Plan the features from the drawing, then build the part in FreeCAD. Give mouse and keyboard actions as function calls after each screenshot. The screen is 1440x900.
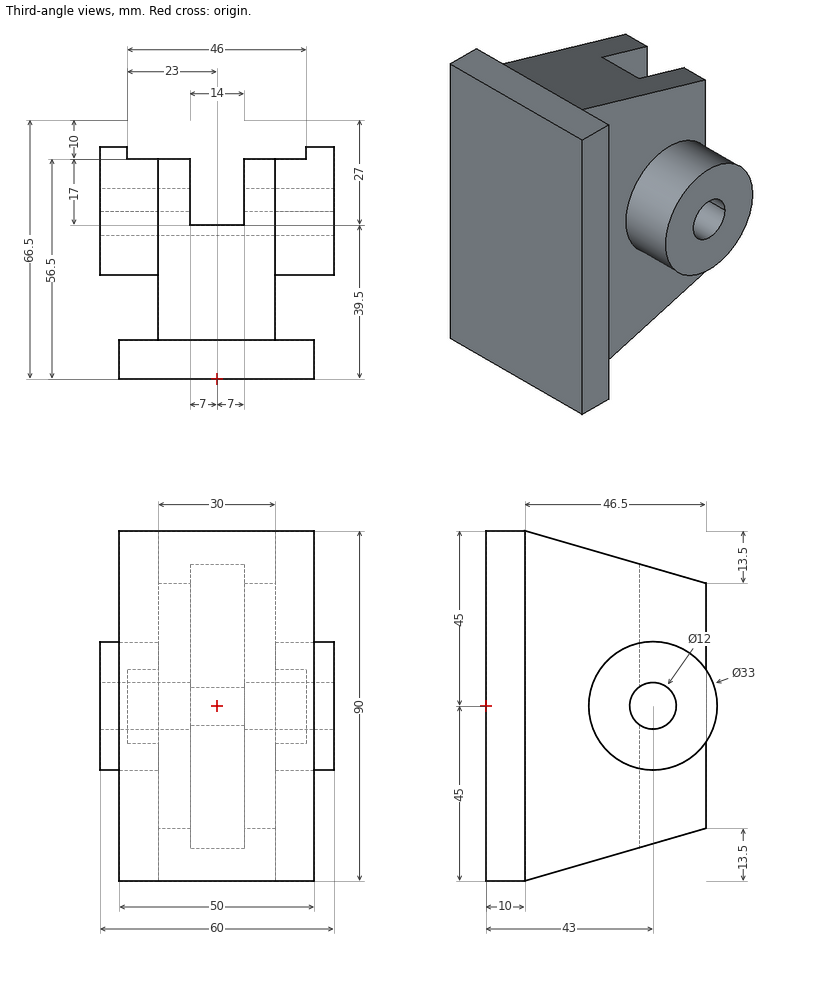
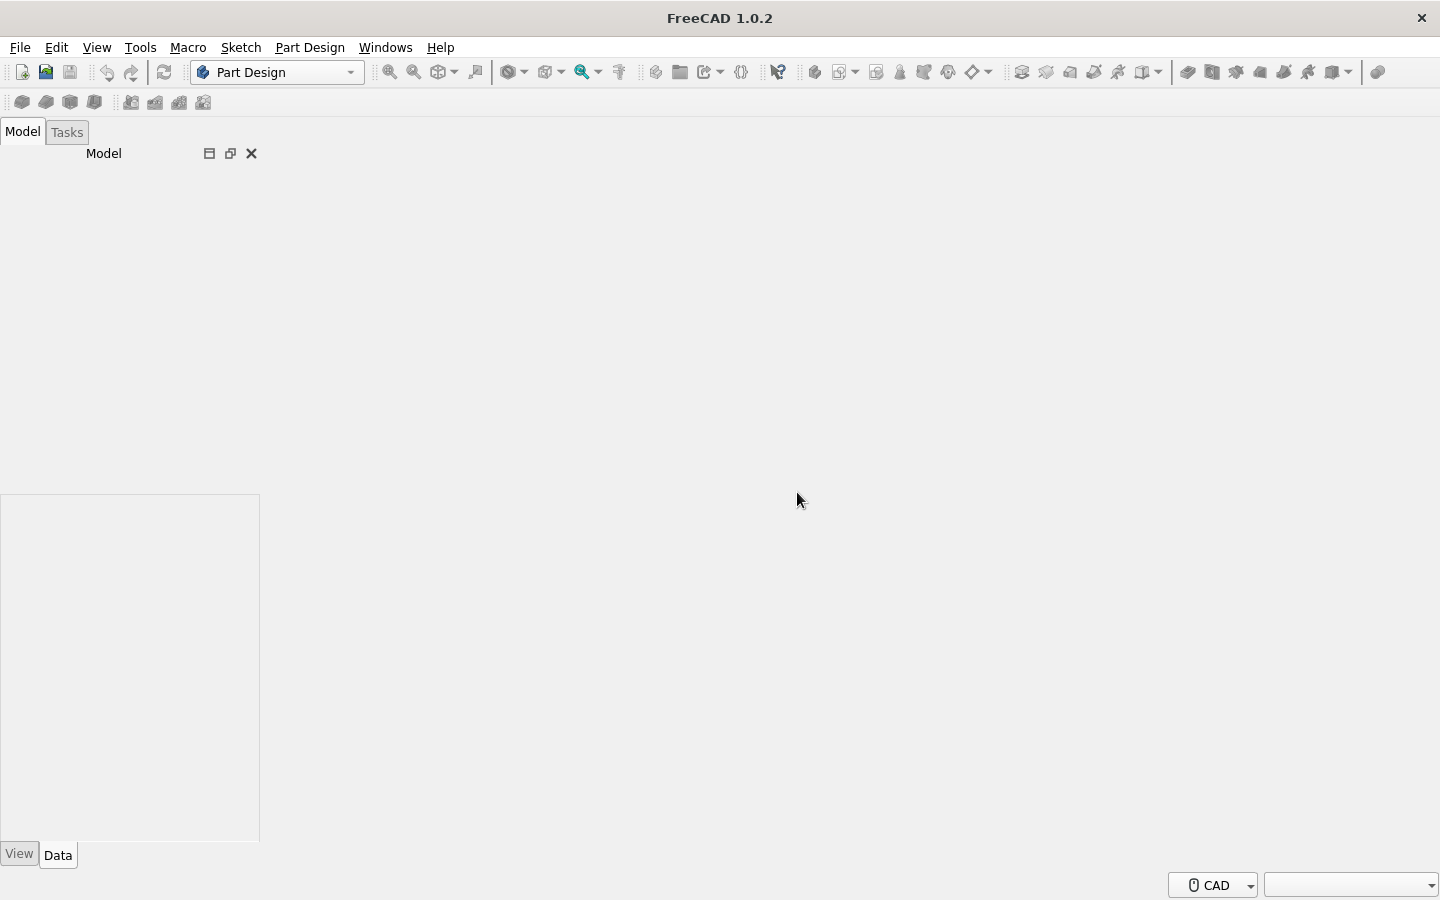
click(22, 72)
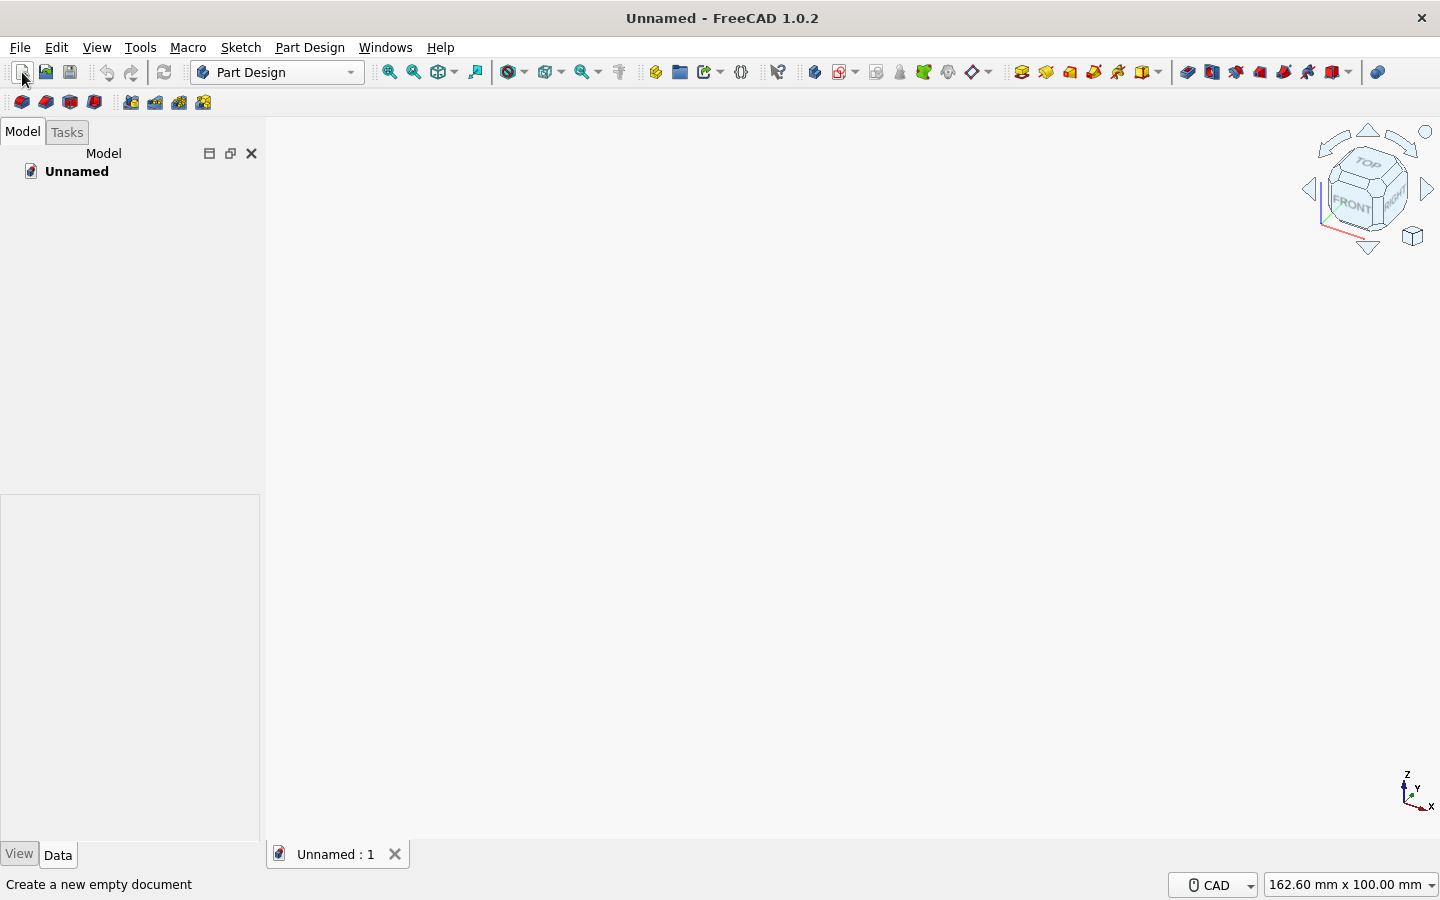
click(840, 72)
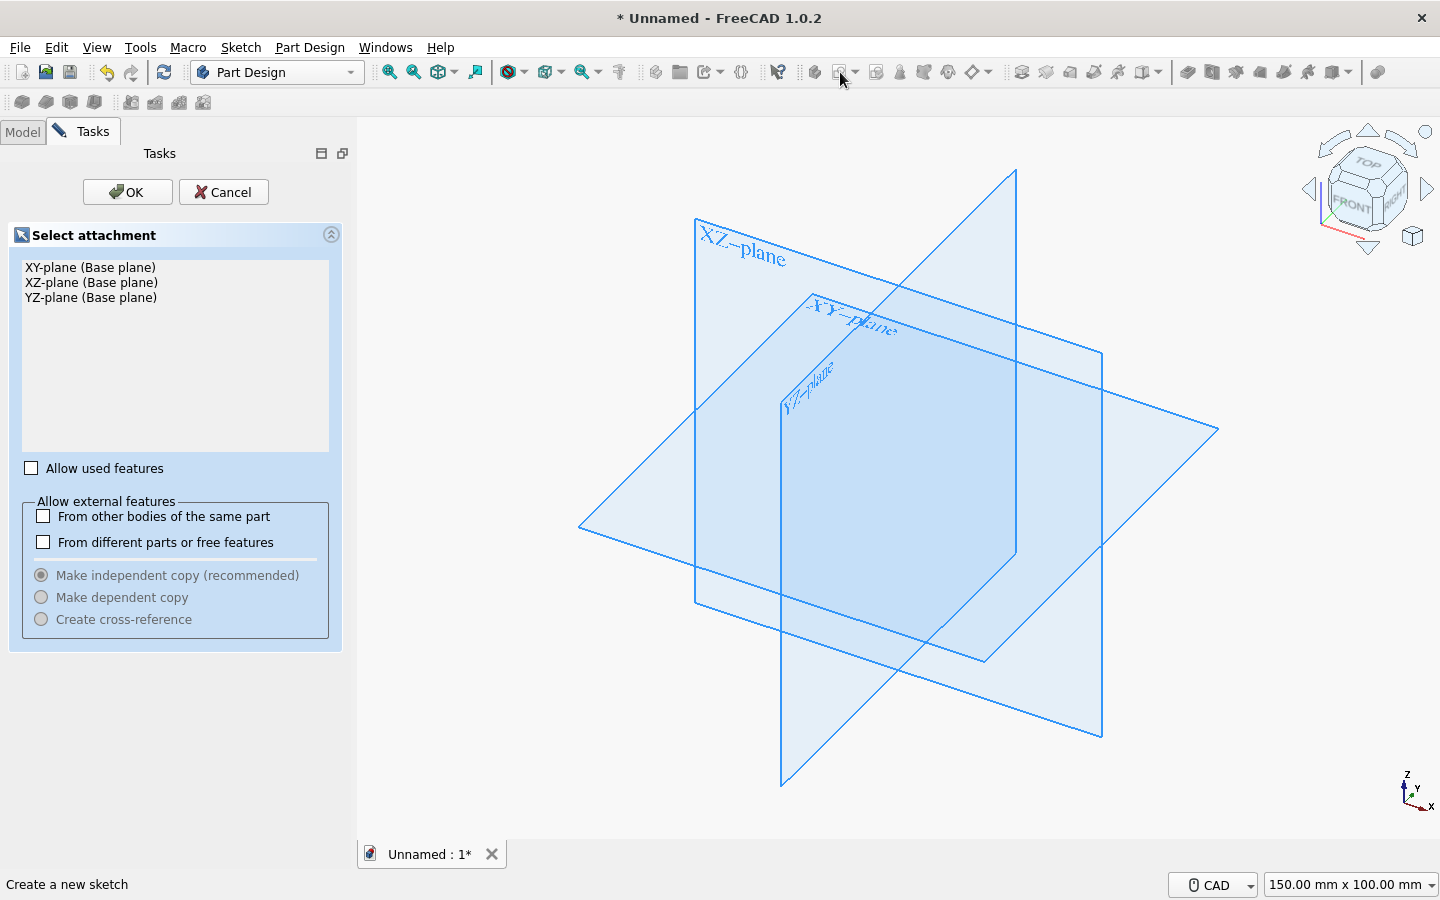
click(82, 282)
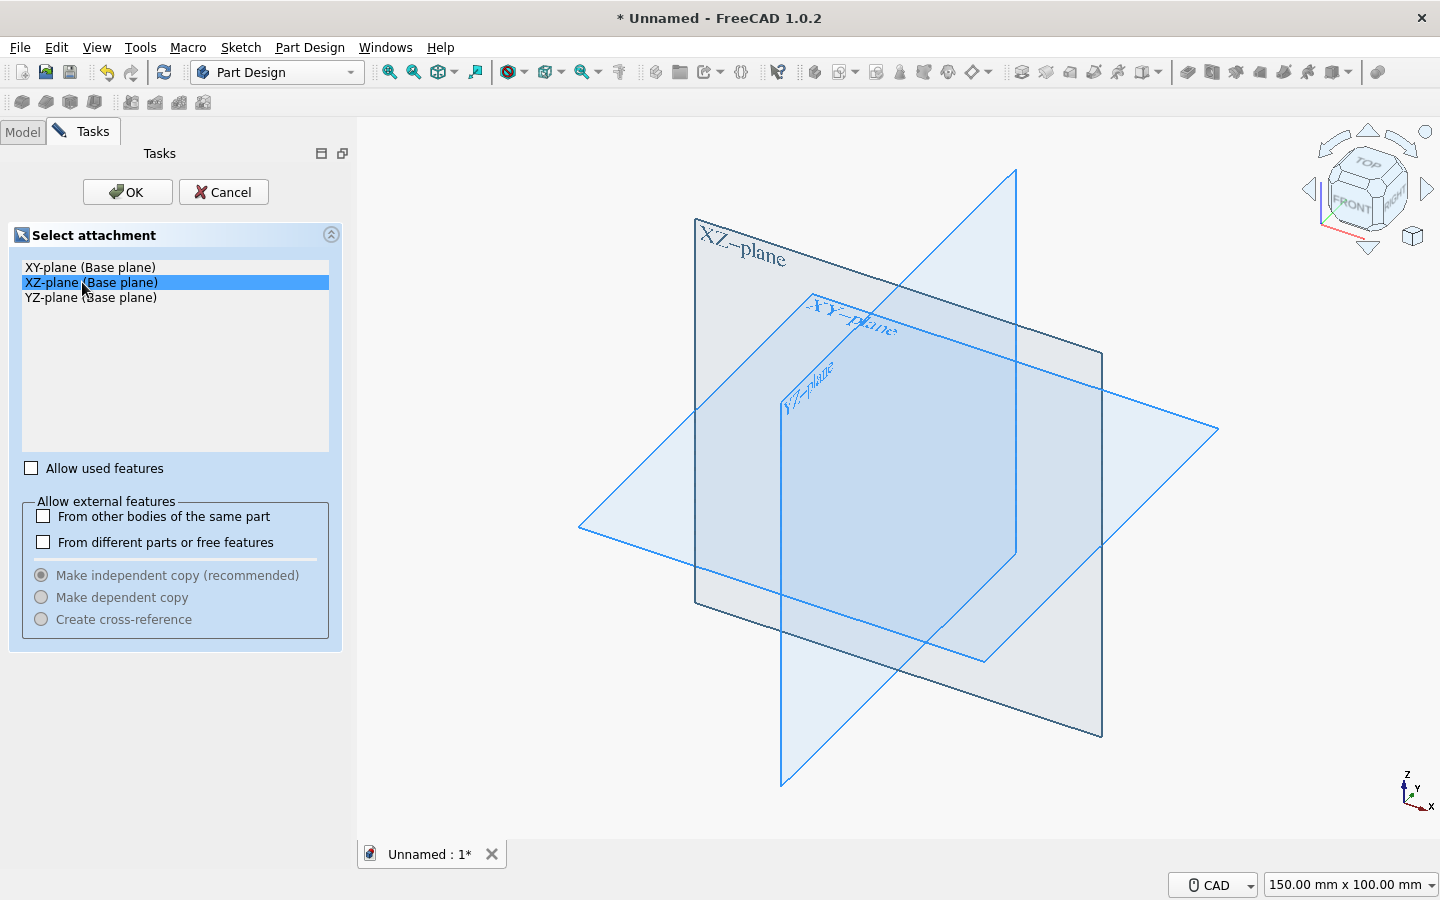
click(128, 192)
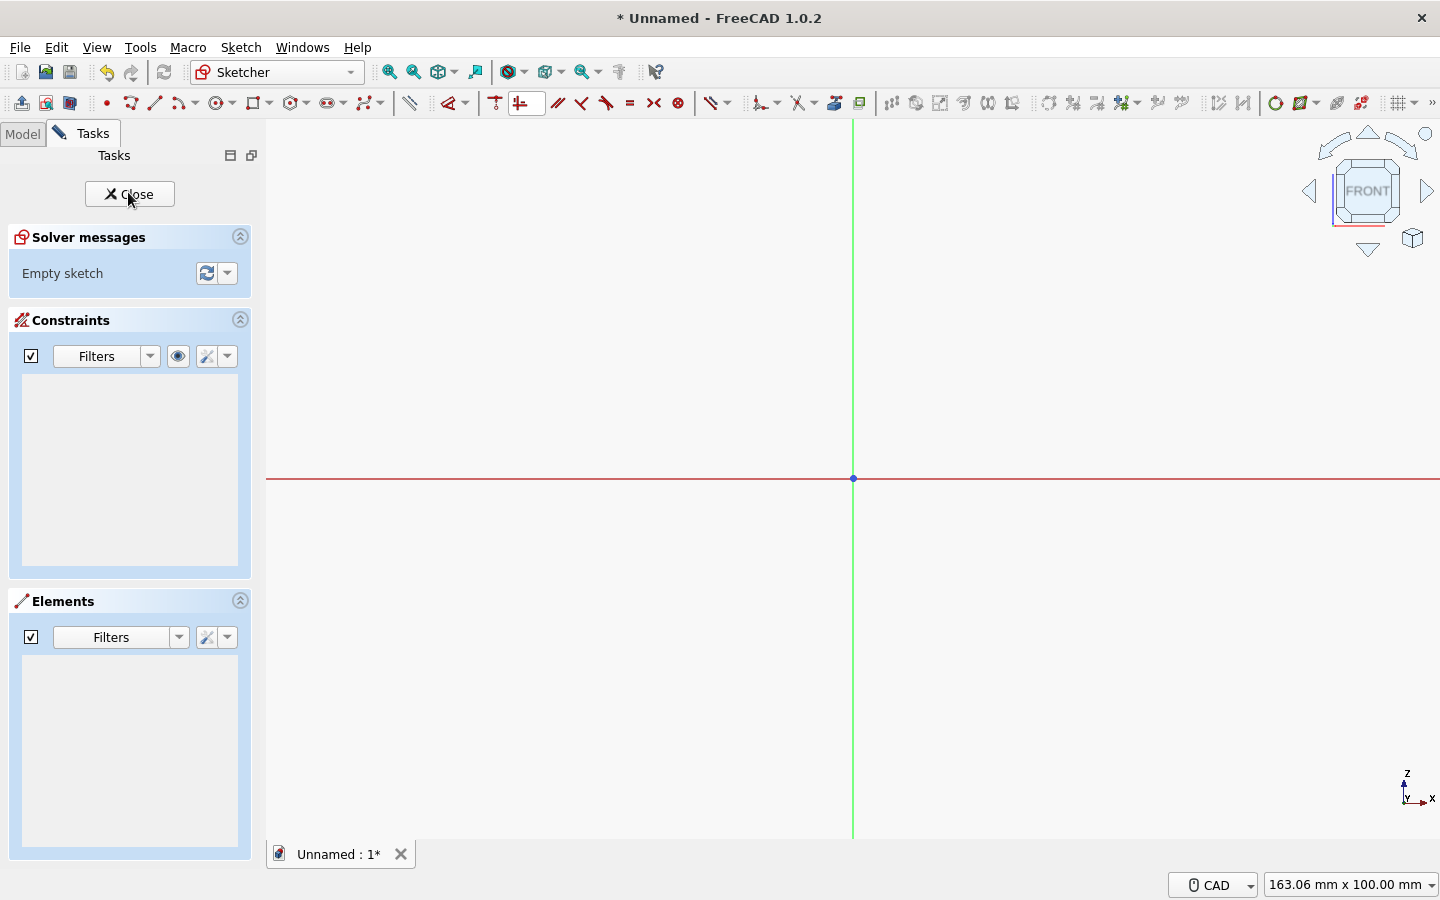
scroll(645, 479, down, 2)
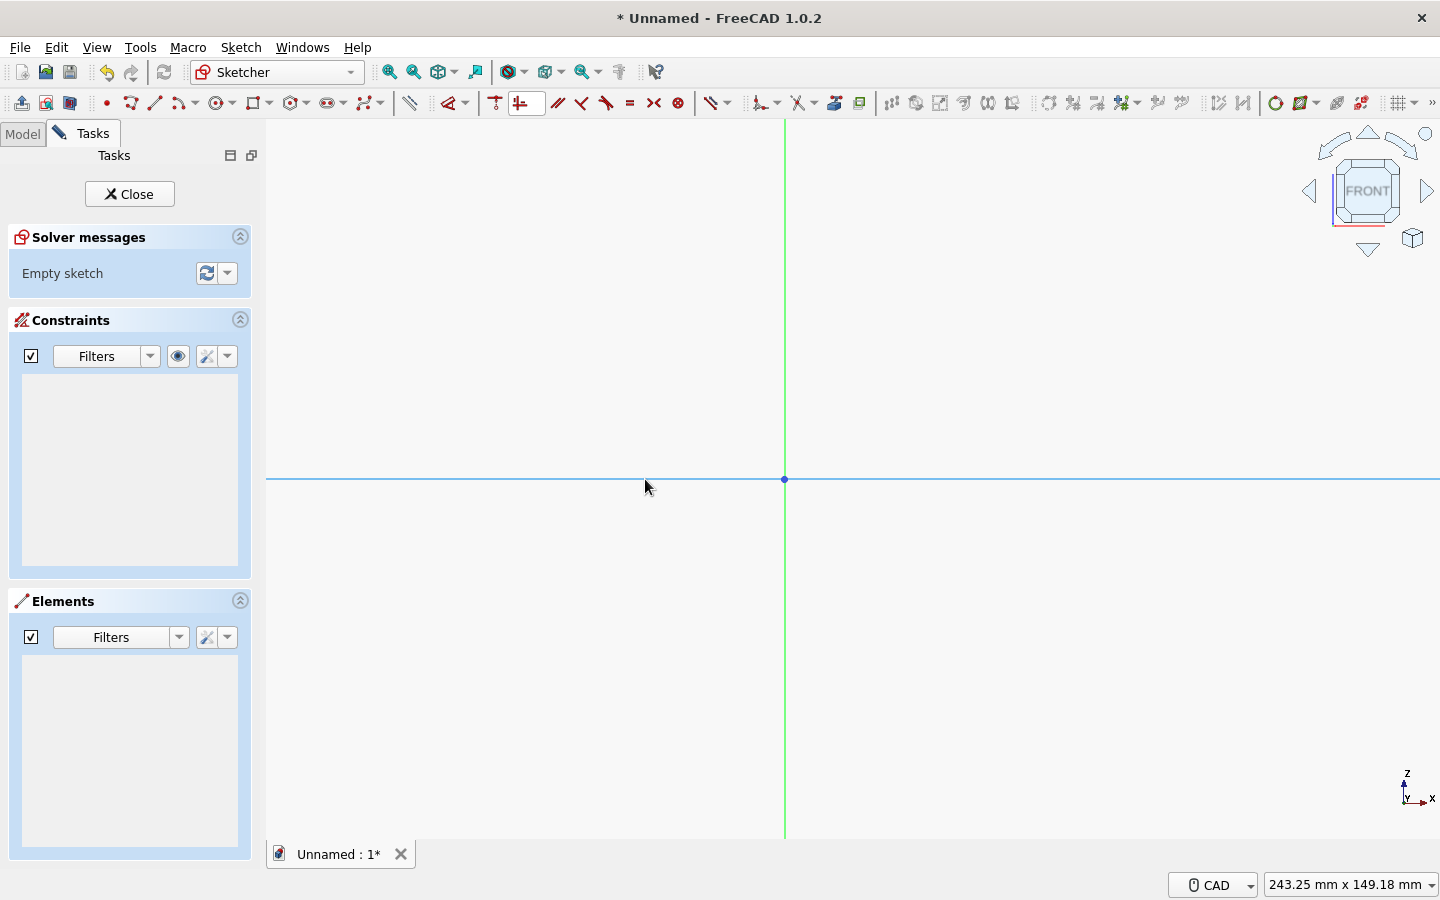
click(272, 104)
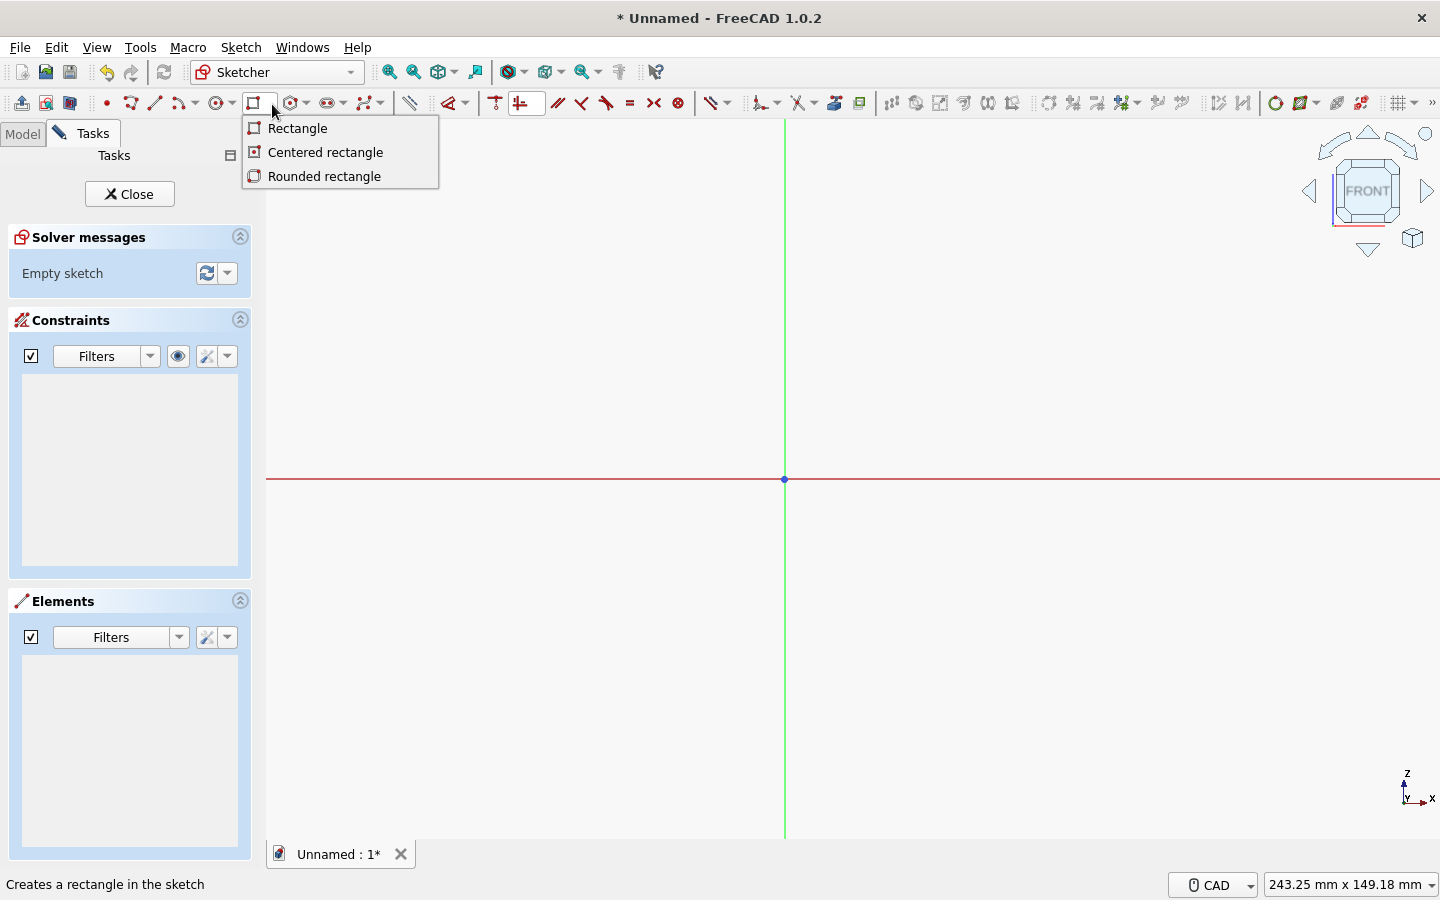
click(340, 152)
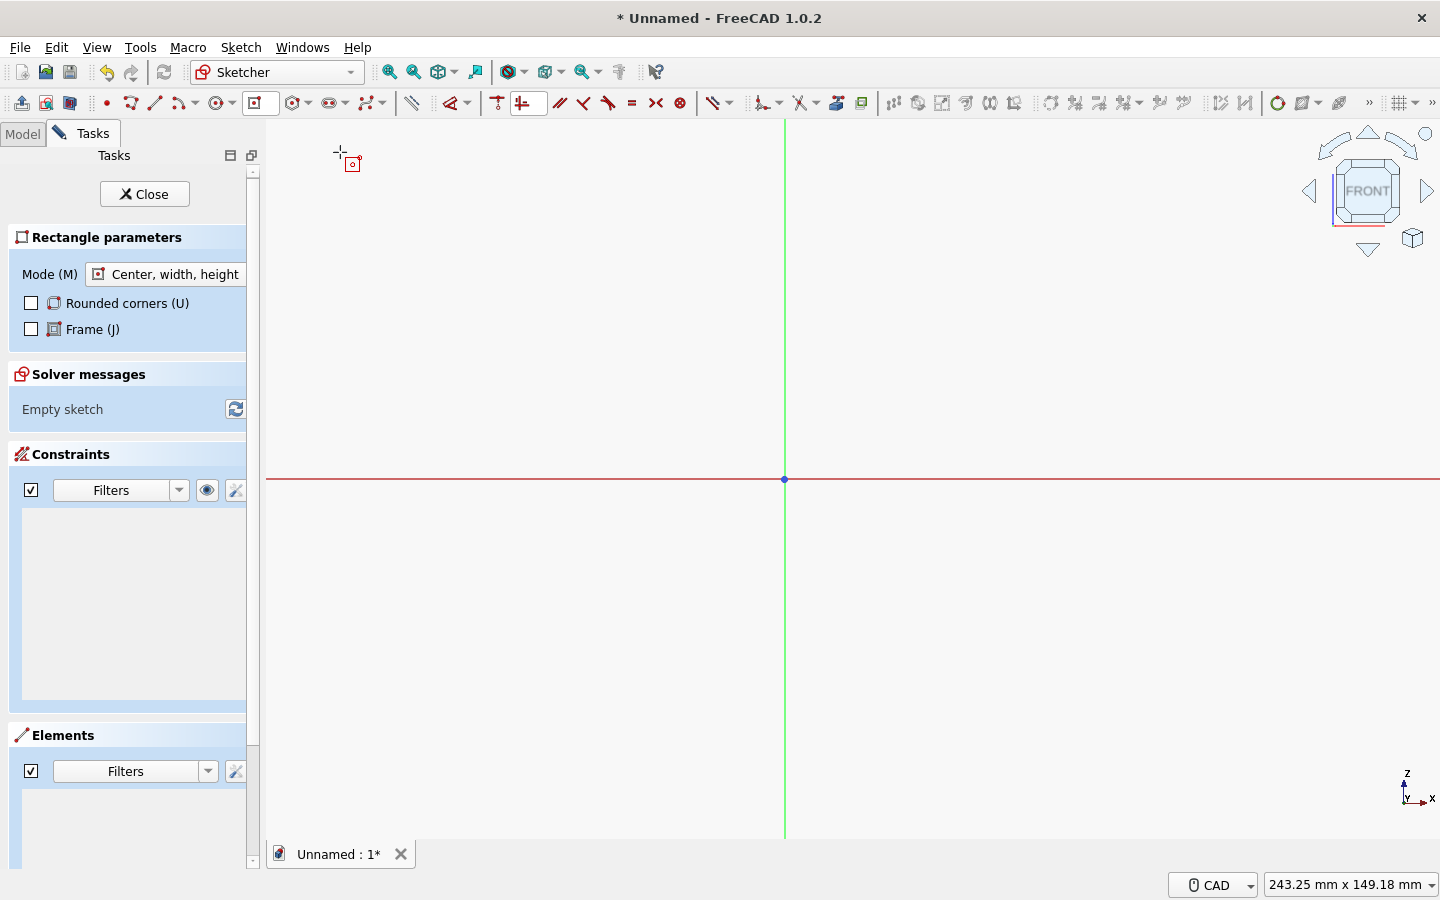
click(785, 479)
click(905, 262)
key(Escape)